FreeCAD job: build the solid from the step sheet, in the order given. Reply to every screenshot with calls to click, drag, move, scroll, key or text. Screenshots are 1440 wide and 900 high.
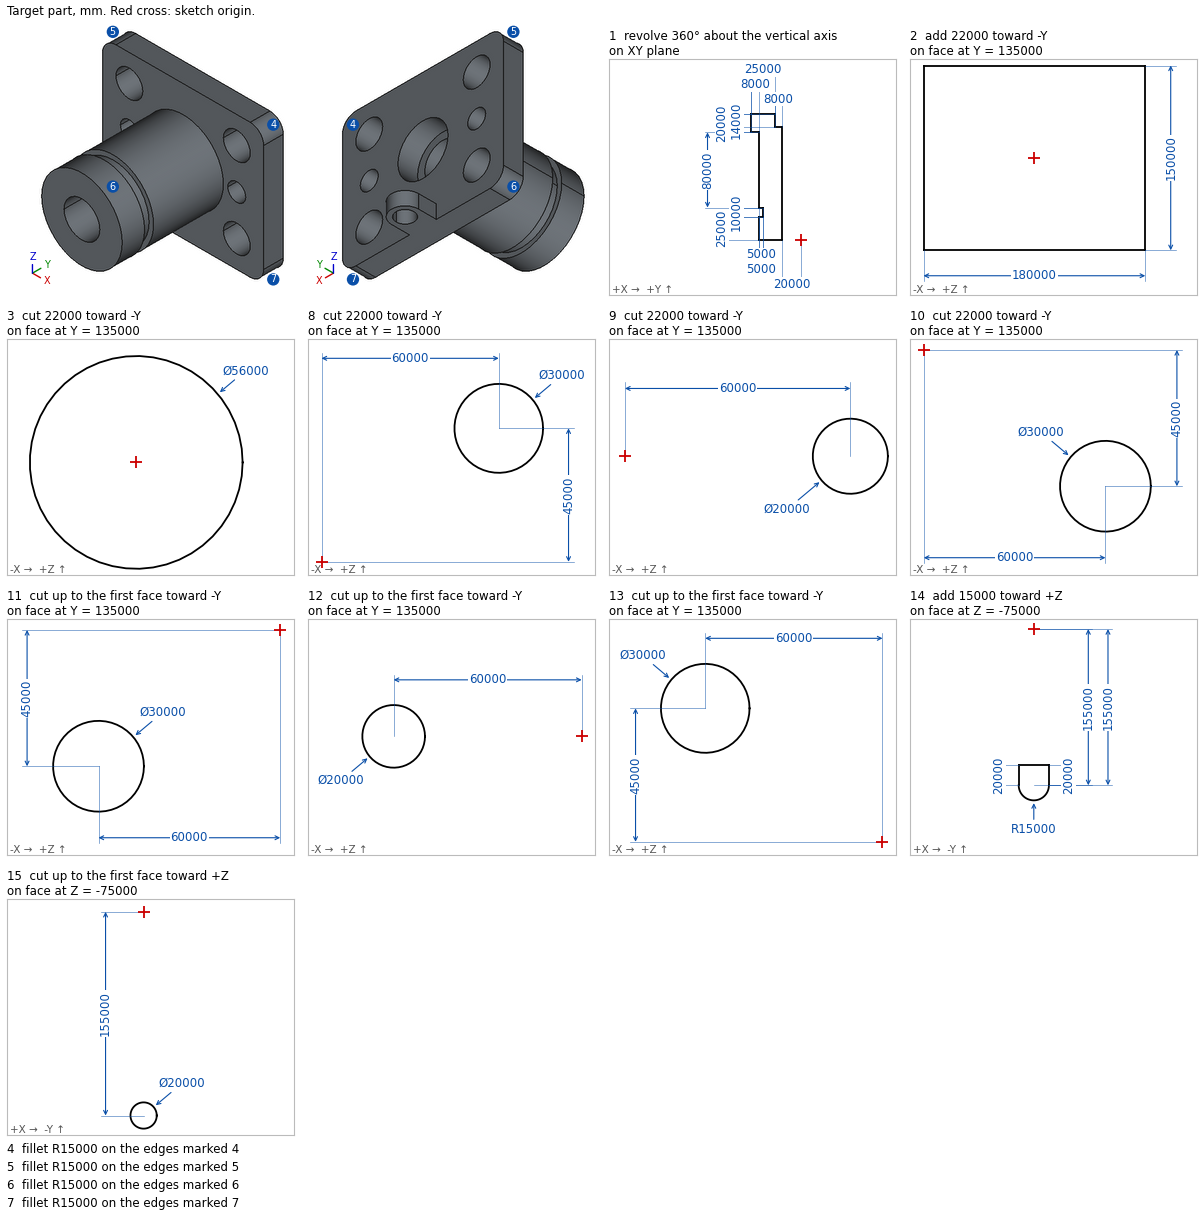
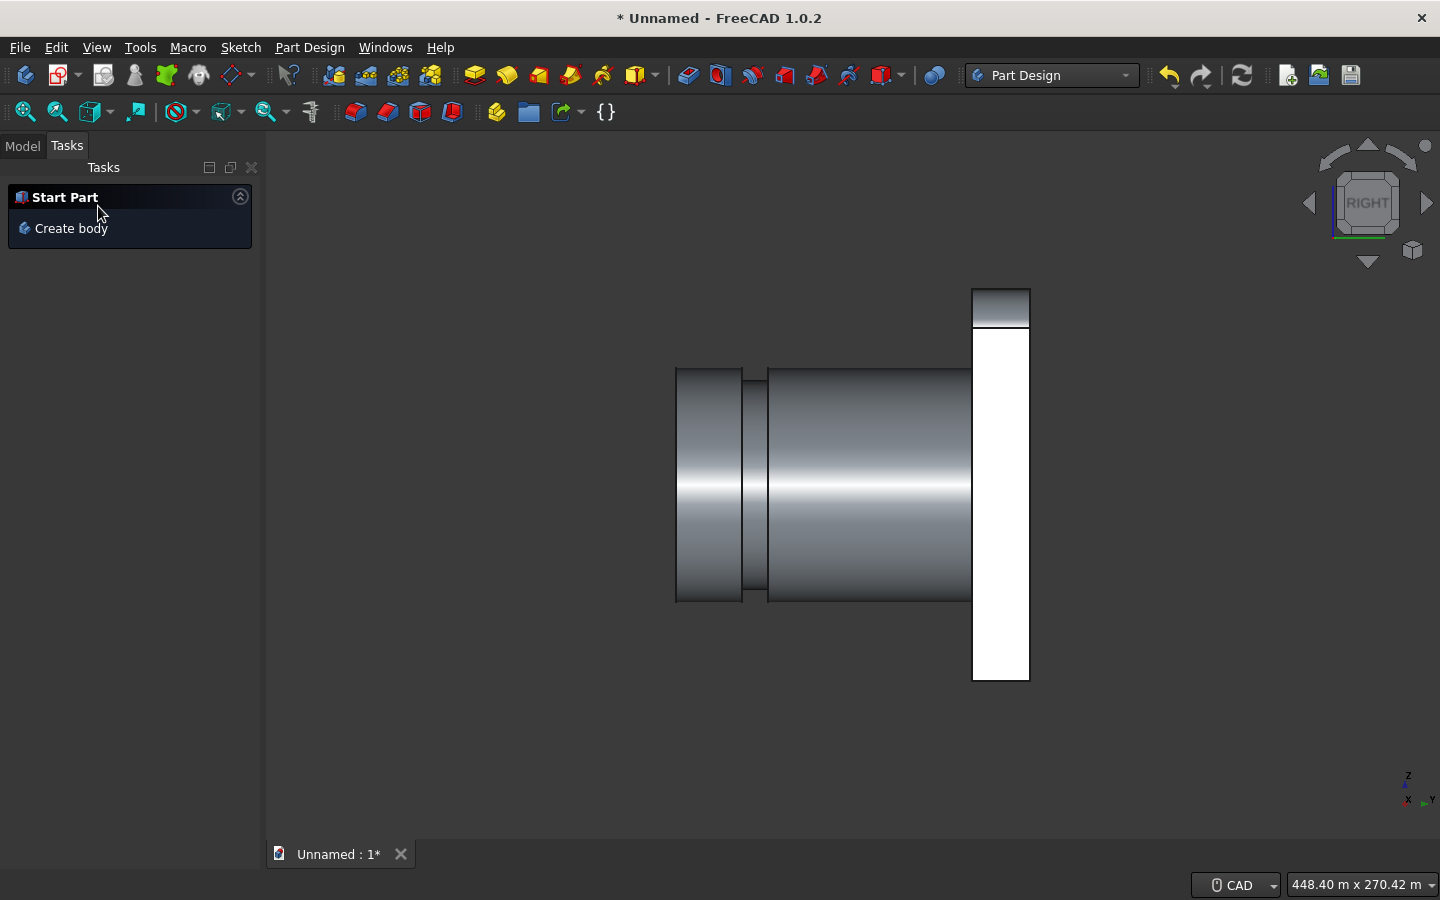
key(5)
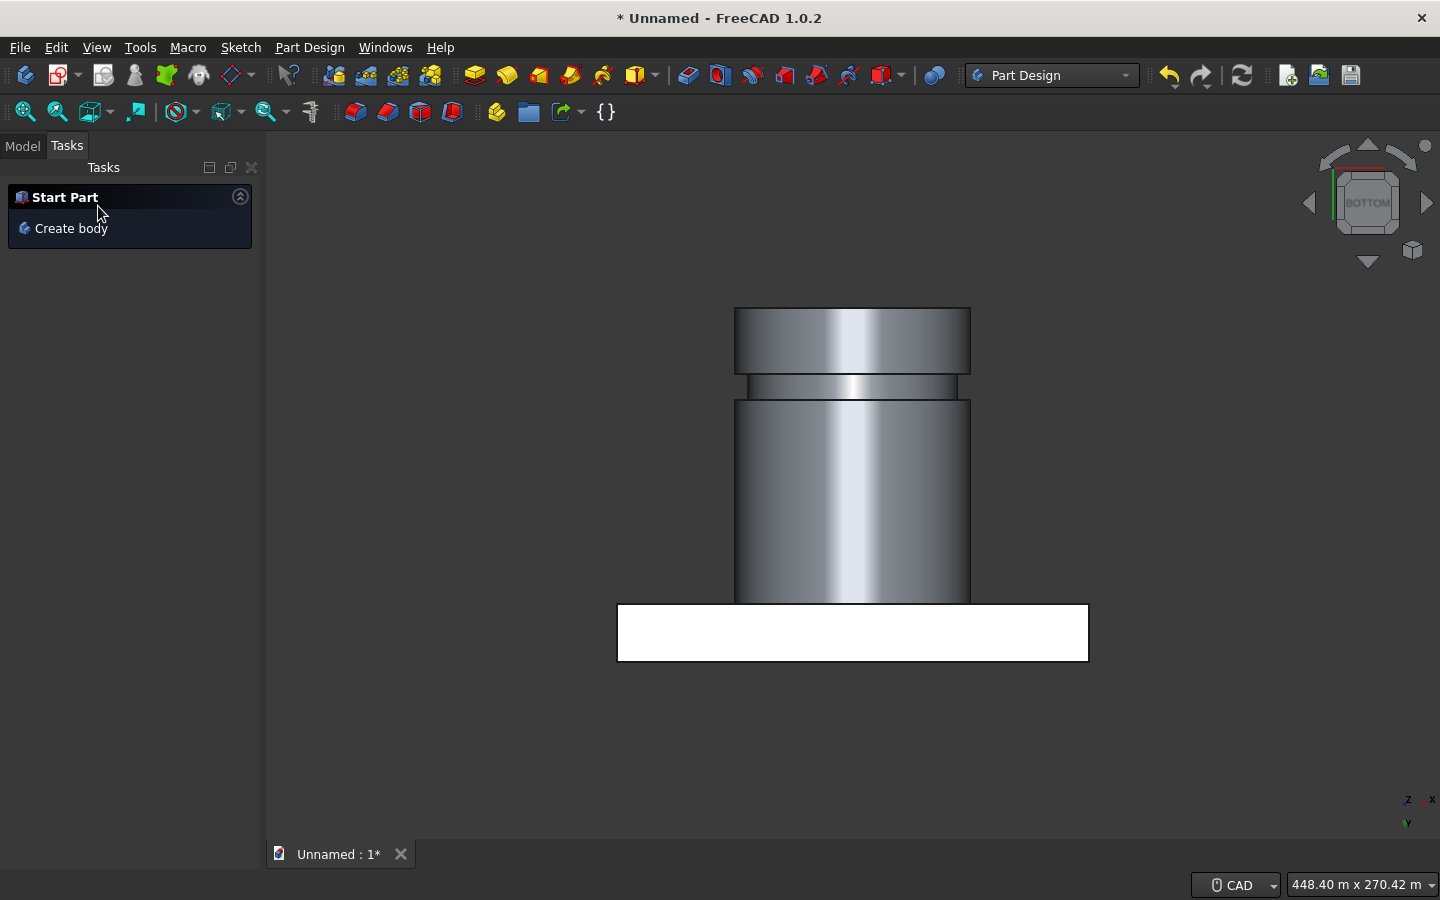
click(617, 632)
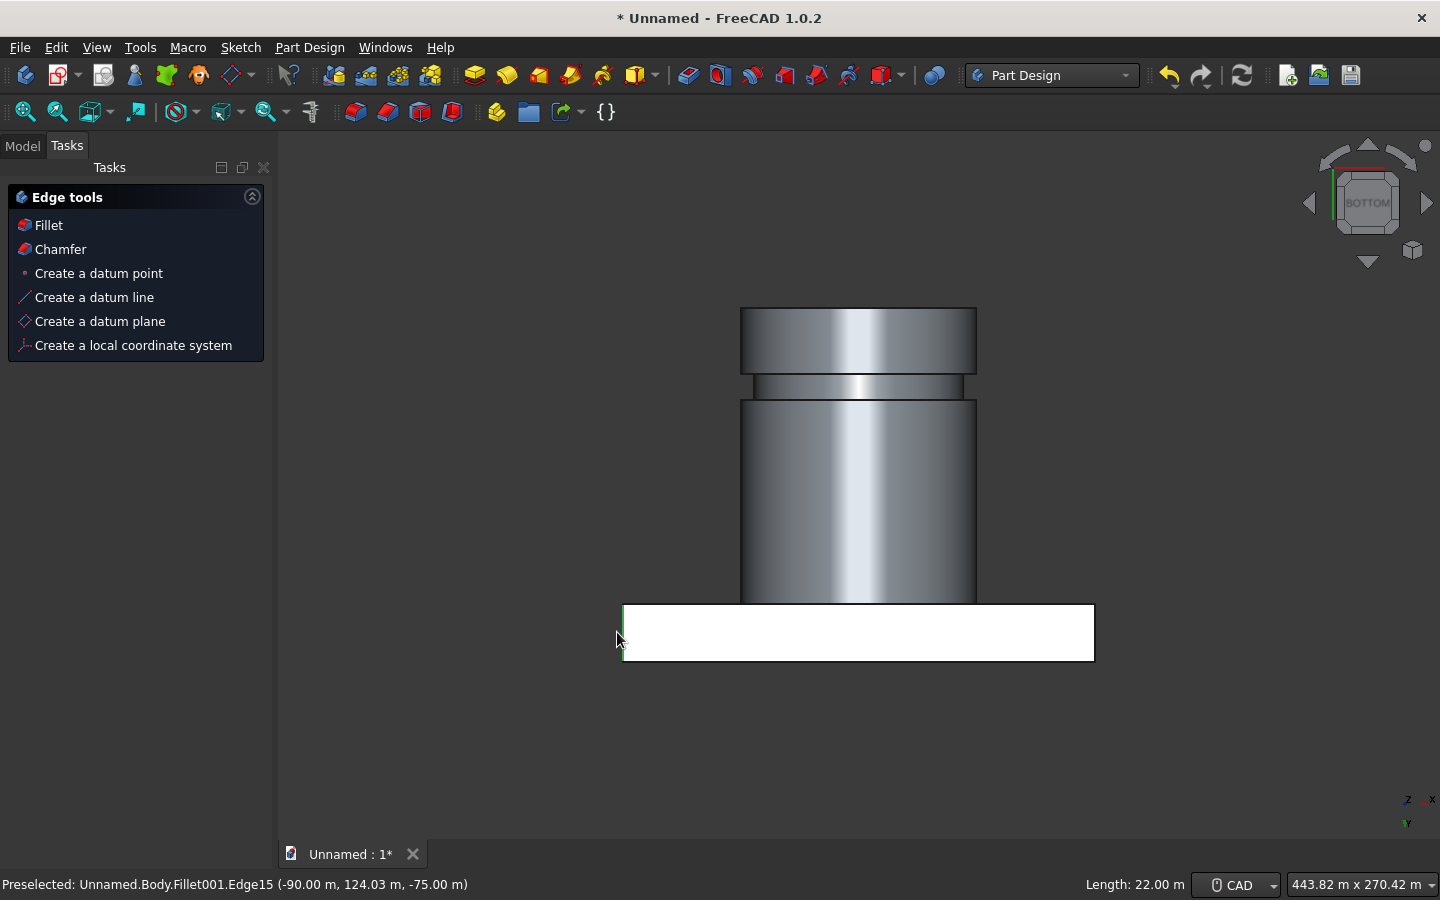
click(356, 112)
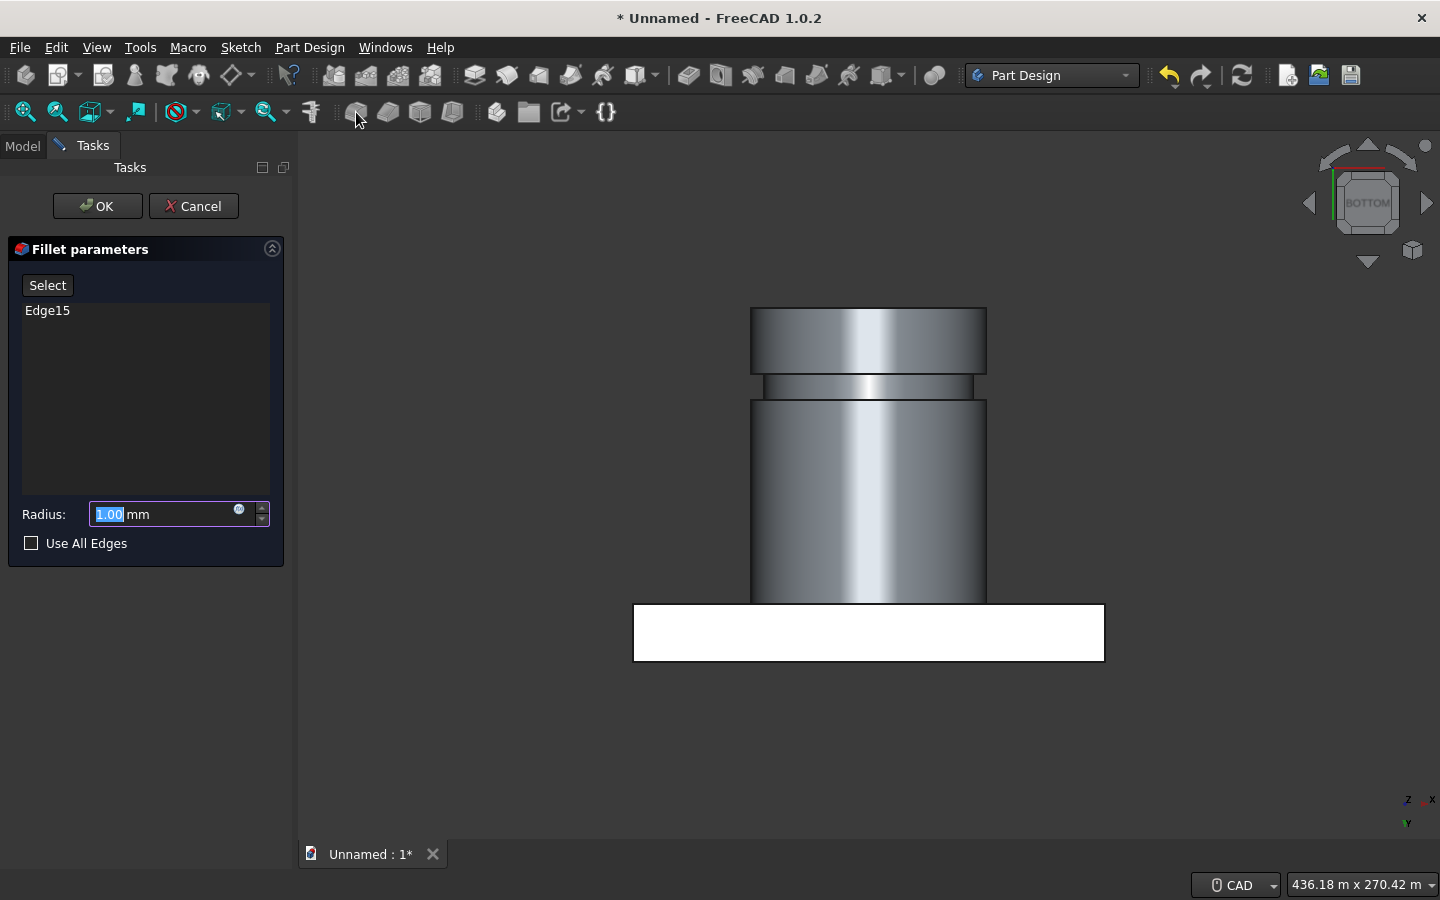
text(15000)
key(Tab)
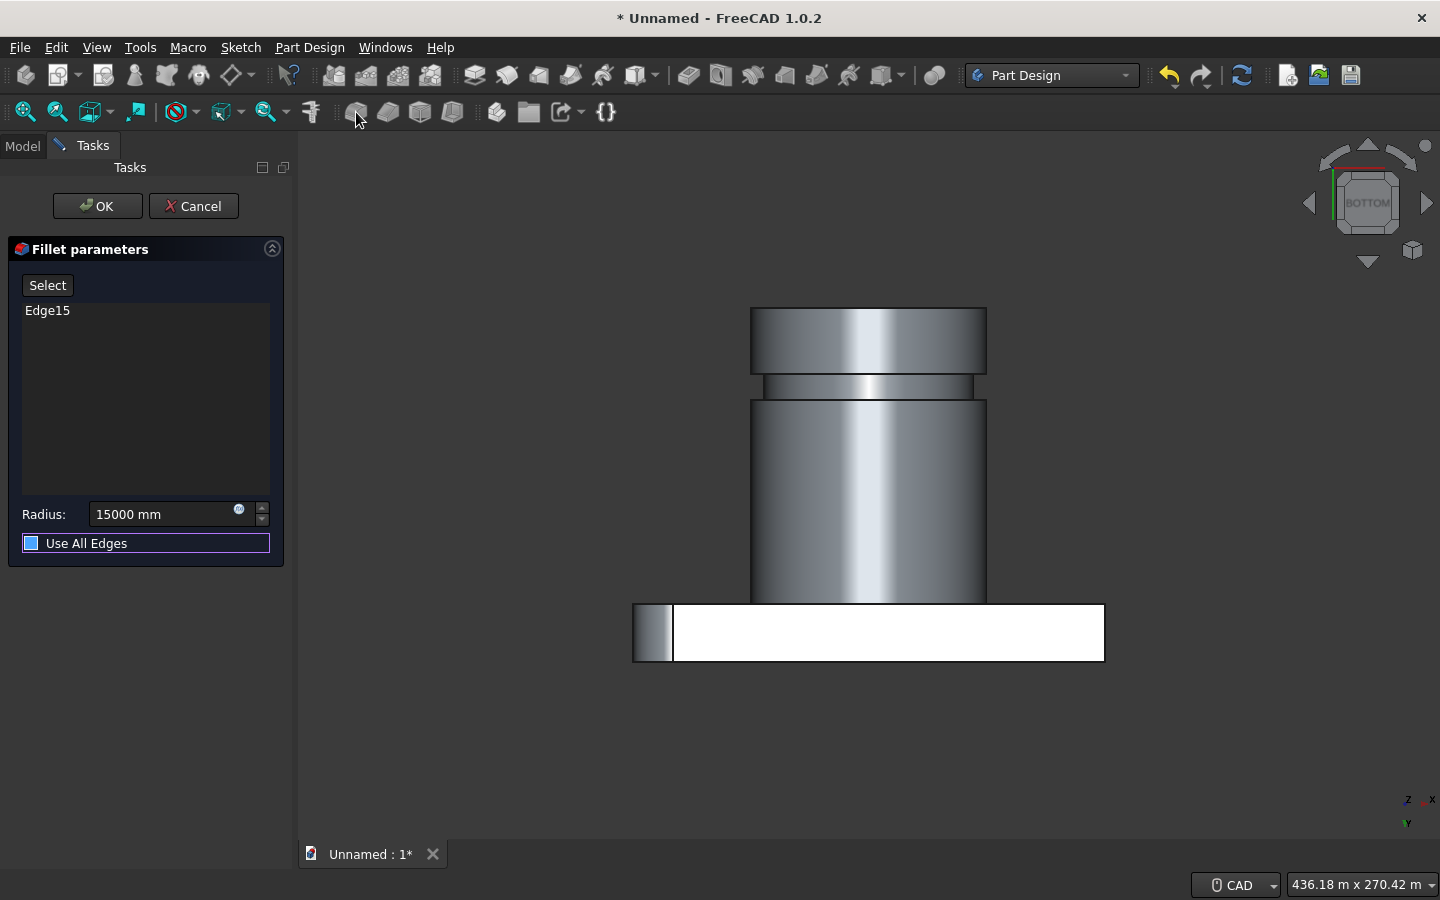
click(98, 206)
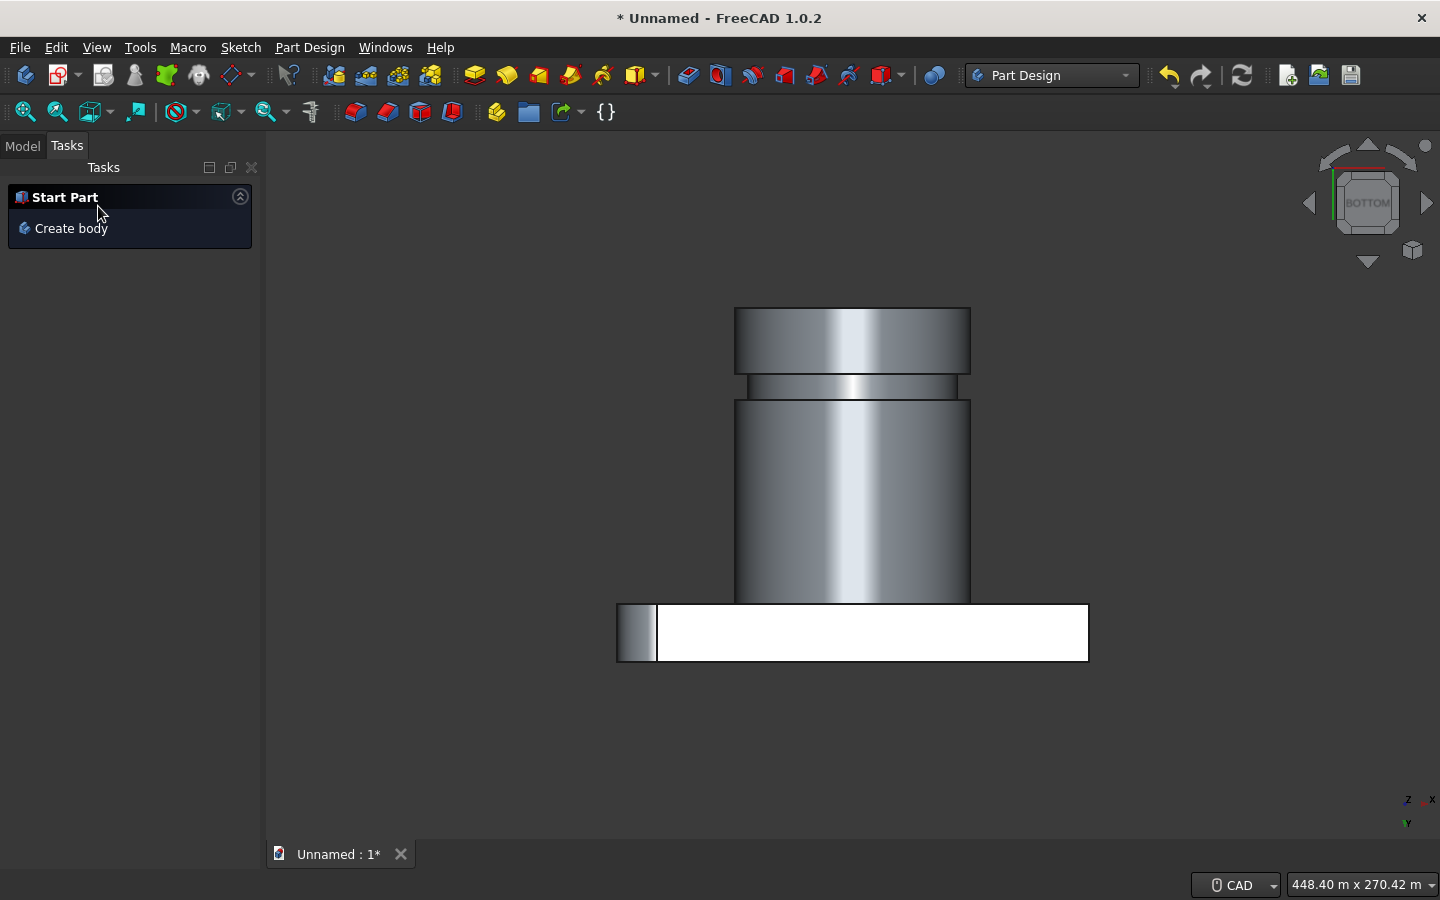
click(1089, 632)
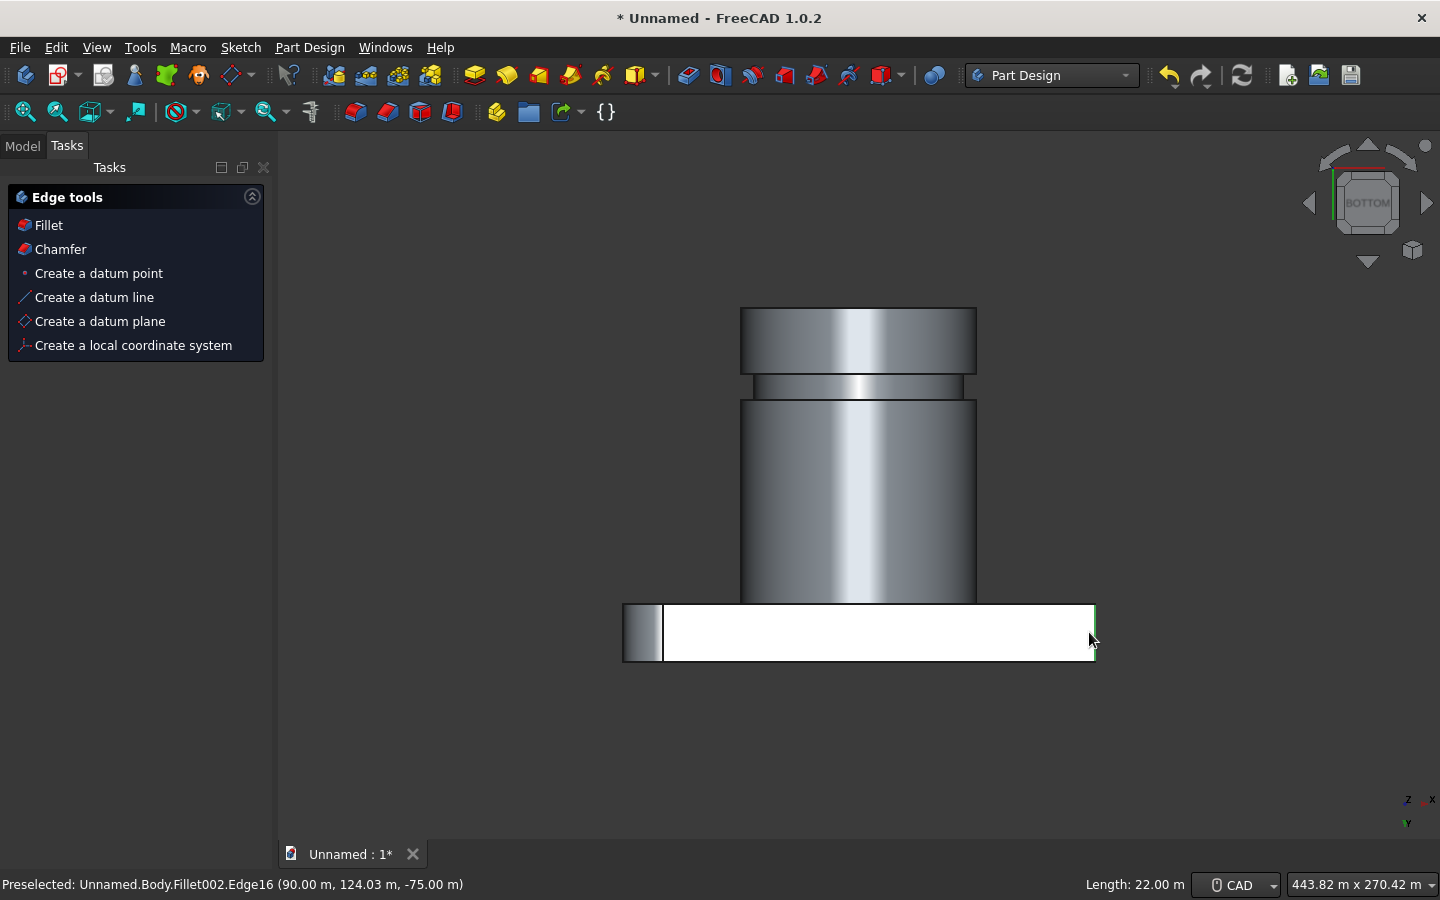
click(356, 112)